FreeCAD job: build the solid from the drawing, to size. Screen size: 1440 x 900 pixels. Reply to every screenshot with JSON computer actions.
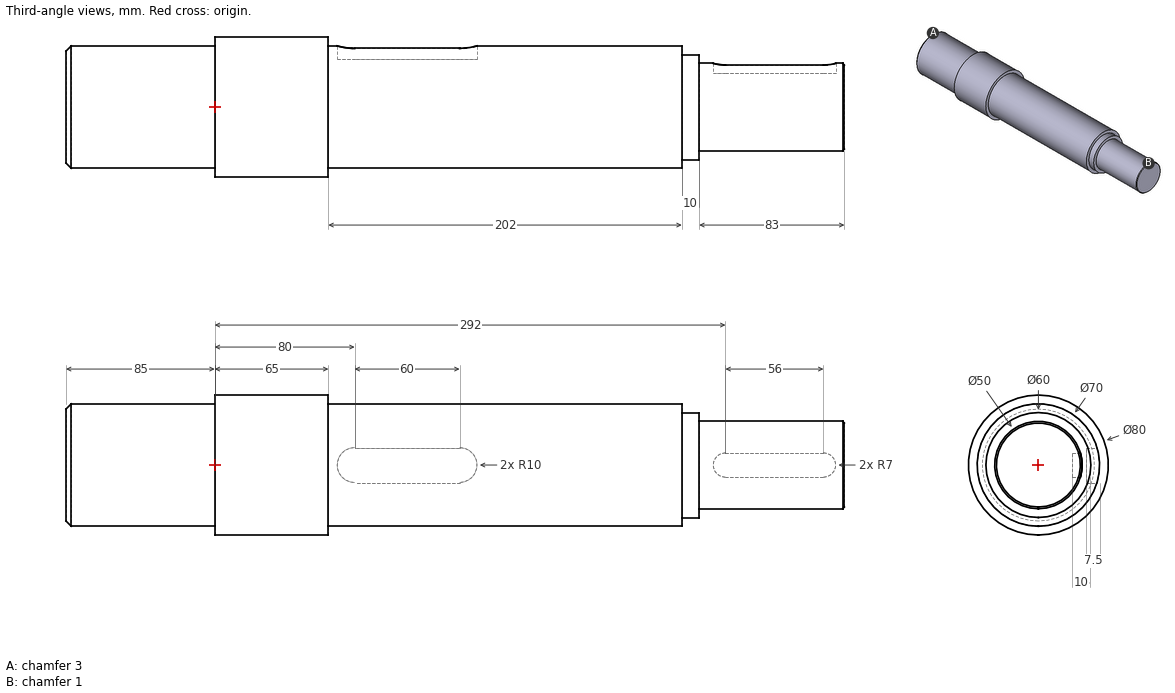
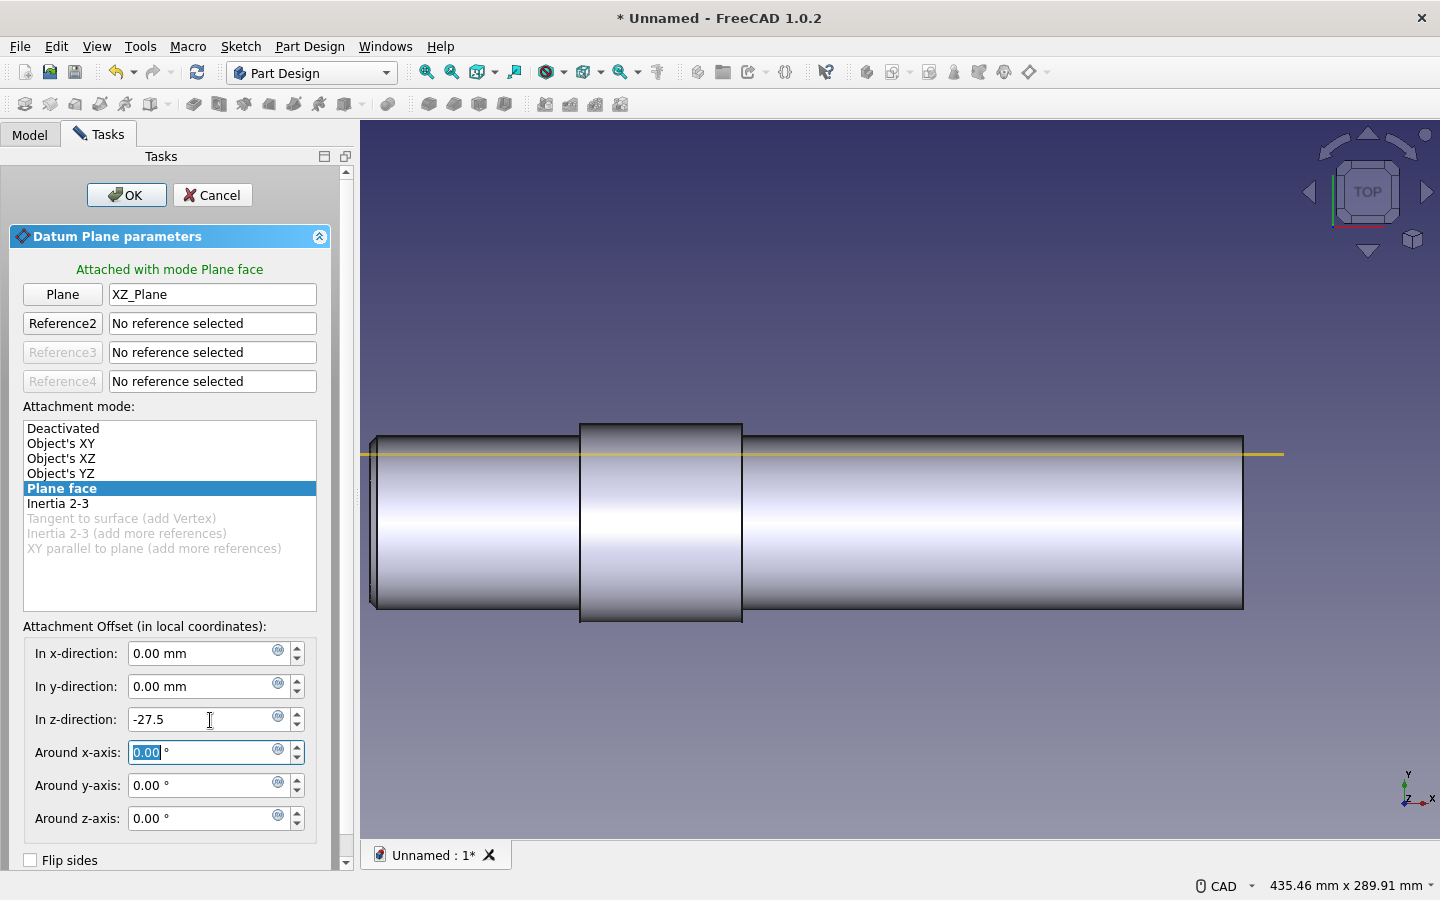
{"action": "left_click", "coordinate": [127, 195]}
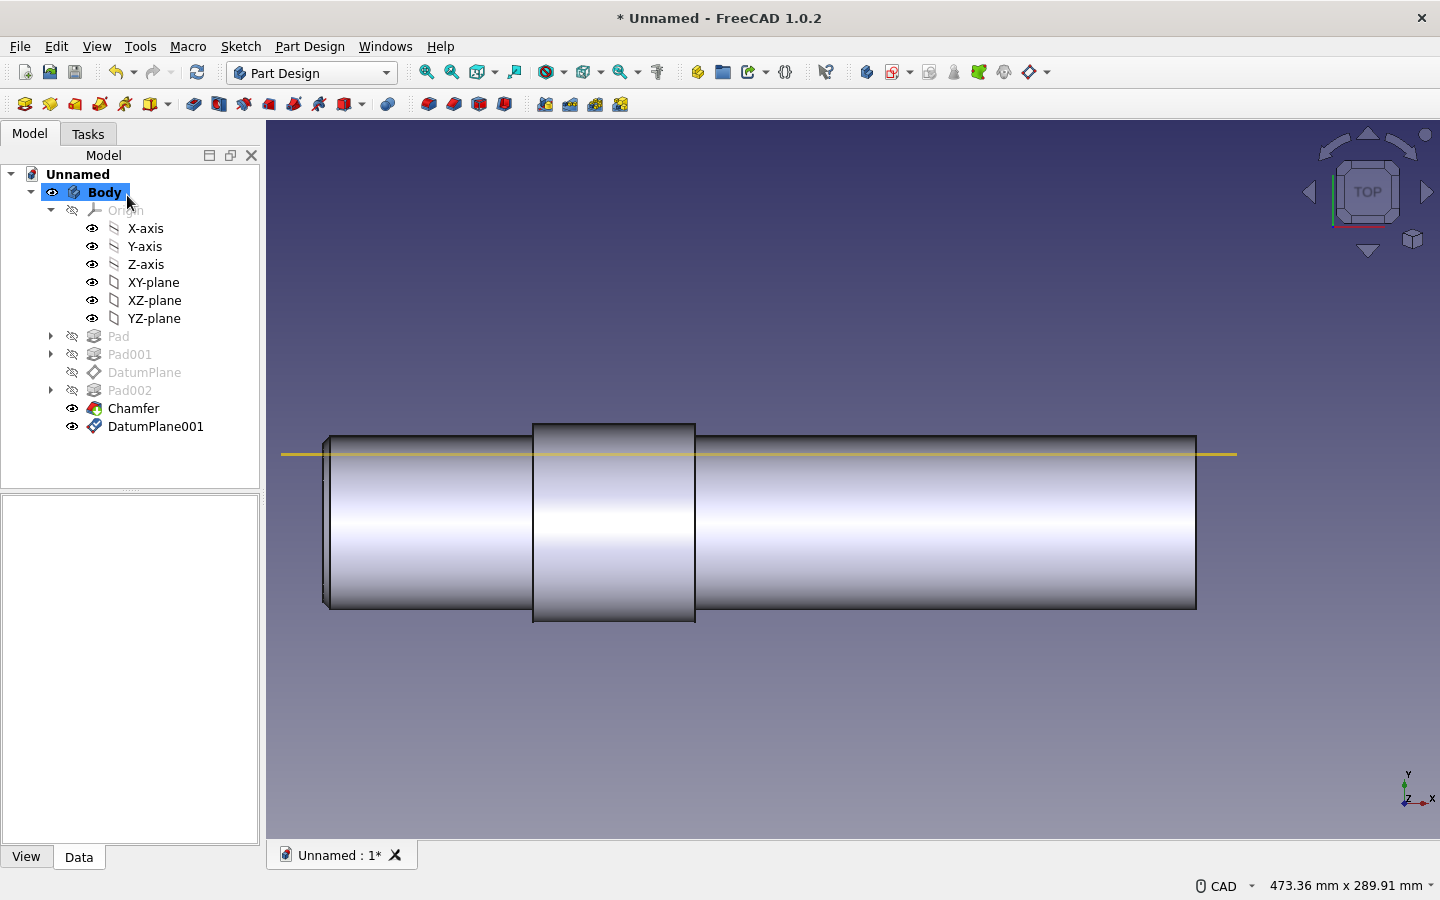
{"action": "left_click", "coordinate": [117, 426]}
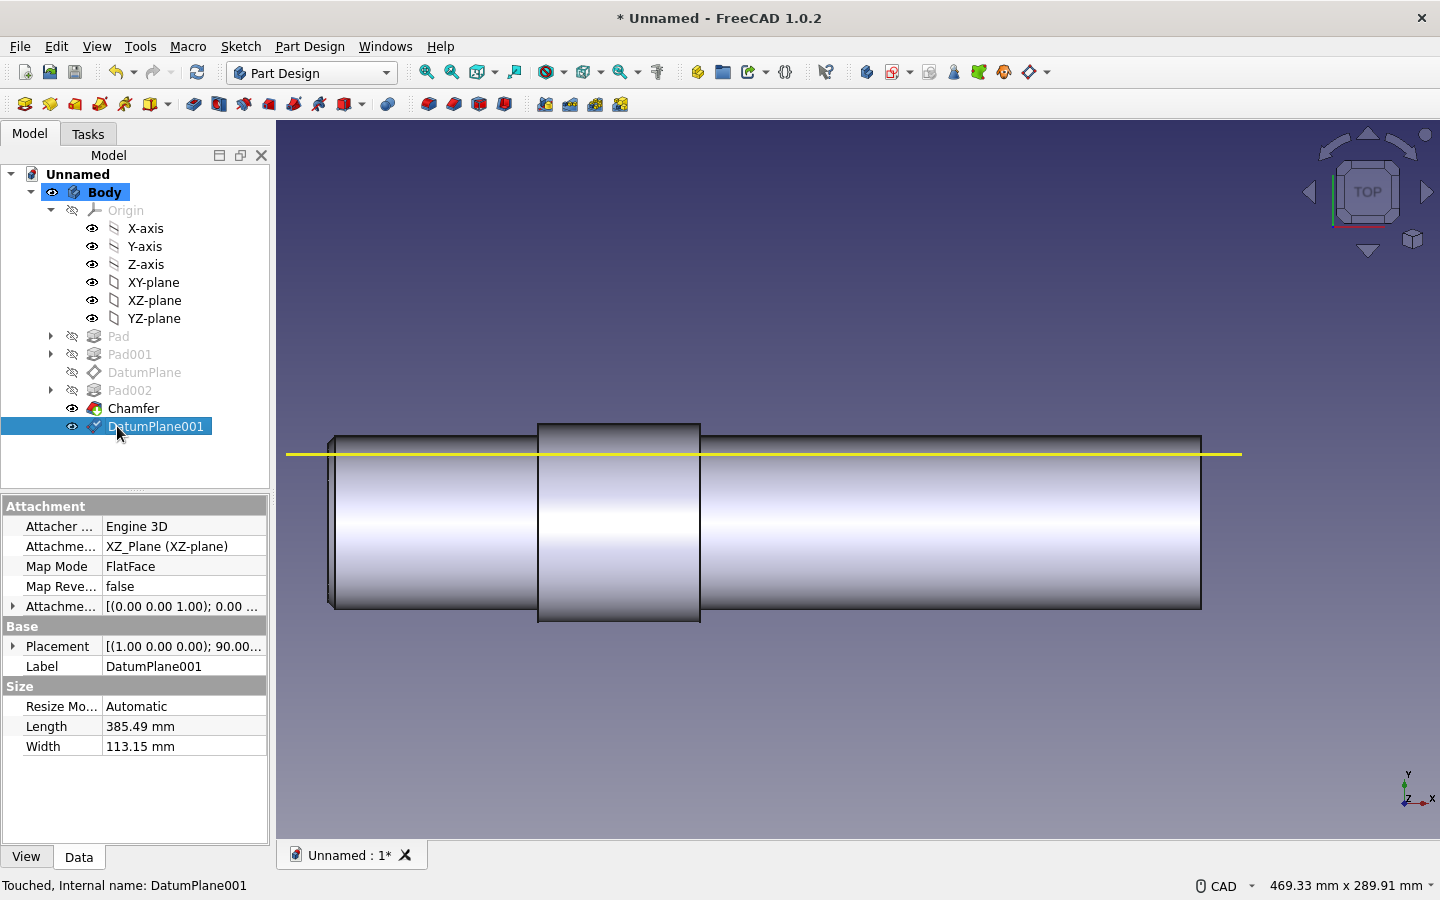
{"action": "left_click", "coordinate": [892, 72]}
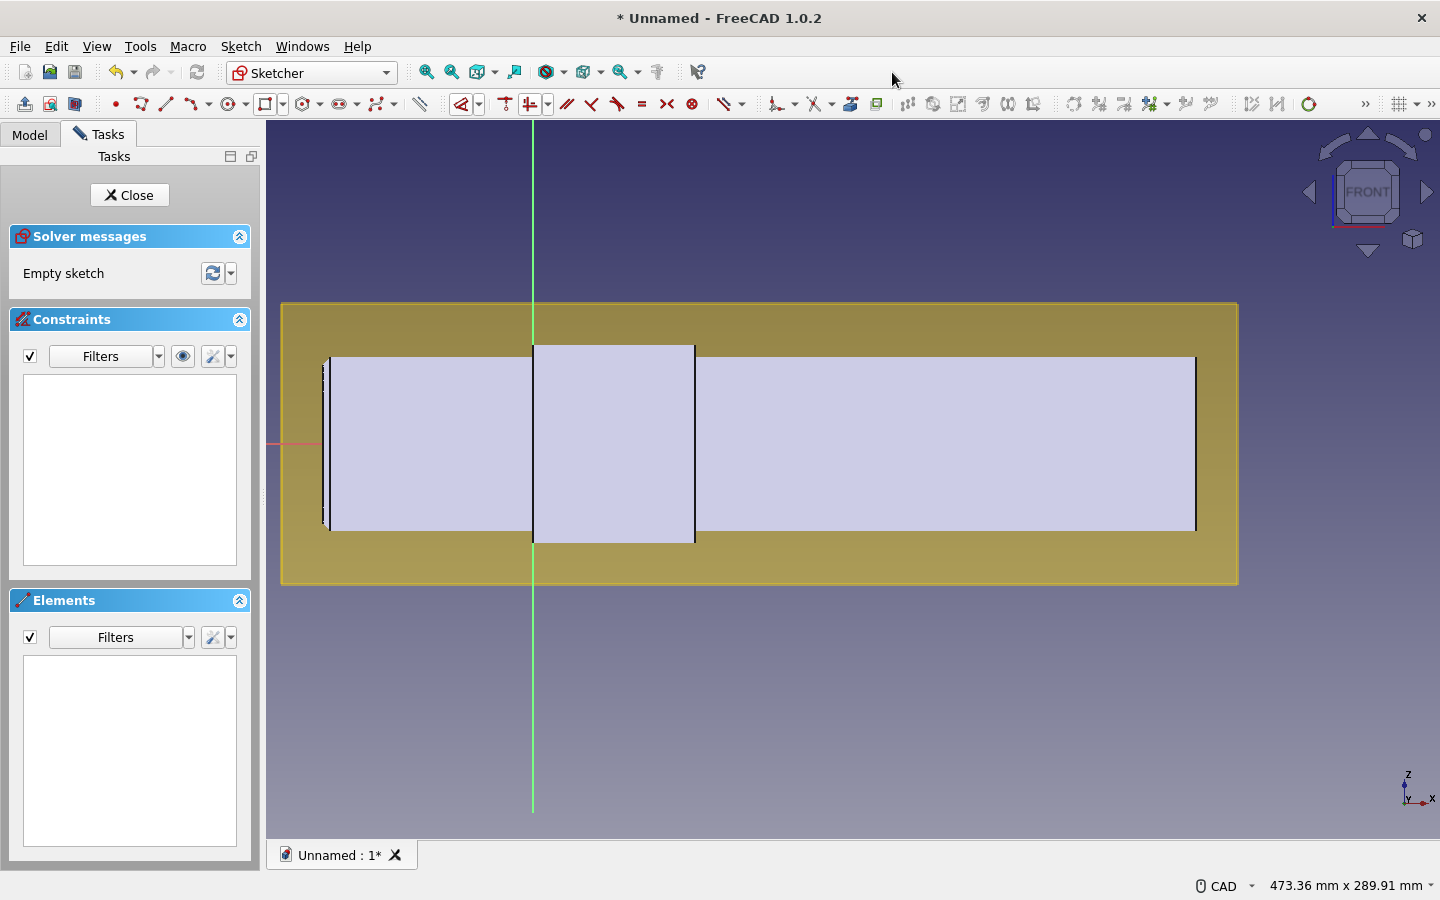
{"action": "left_click", "coordinate": [75, 104]}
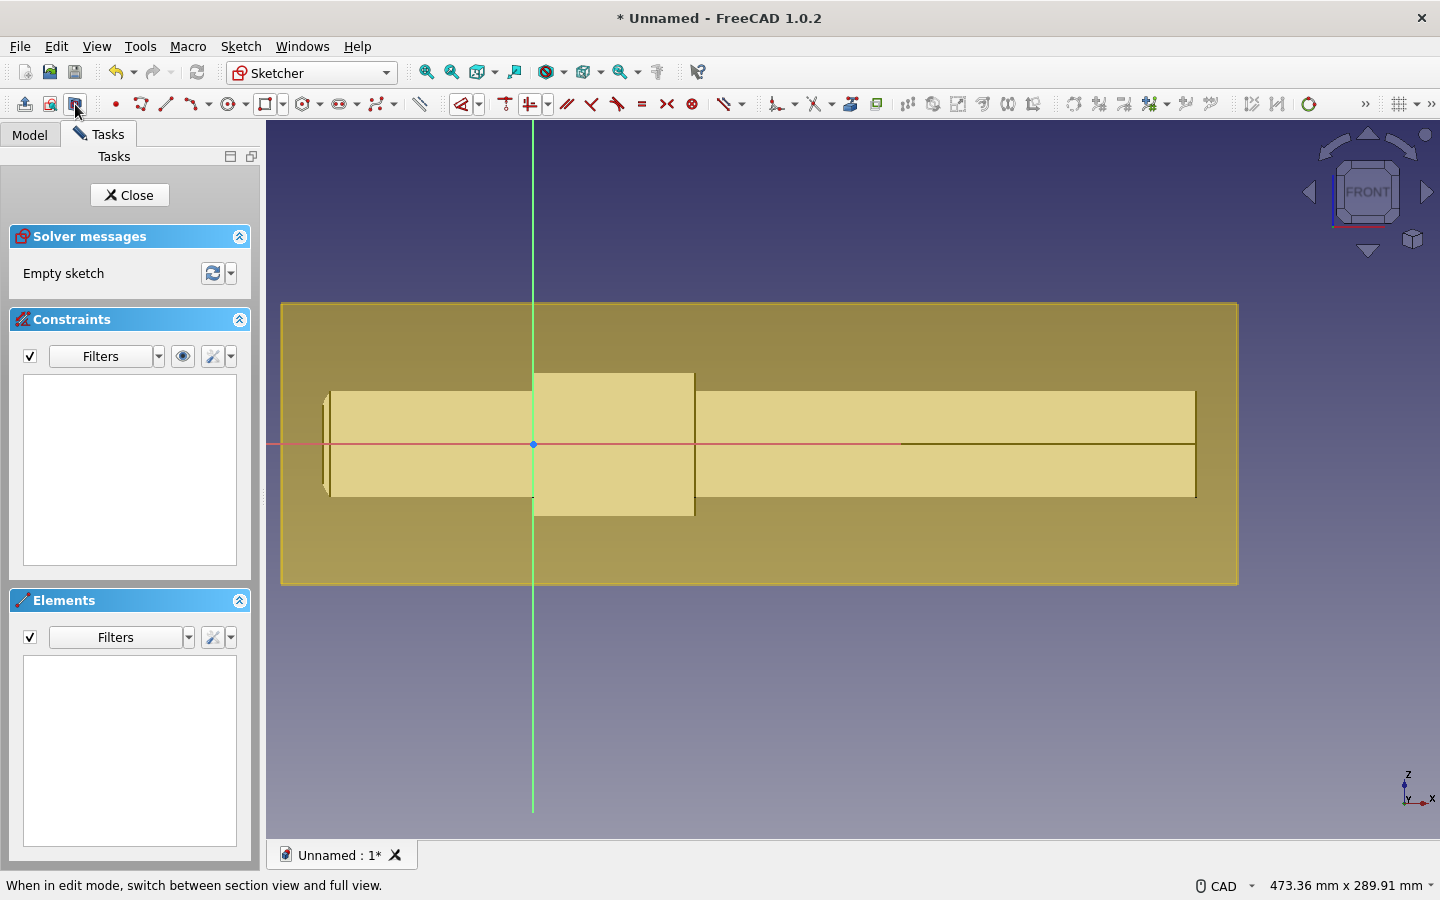
{"action": "scroll", "coordinate": [640, 401], "scroll_direction": "up", "scroll_amount": 3}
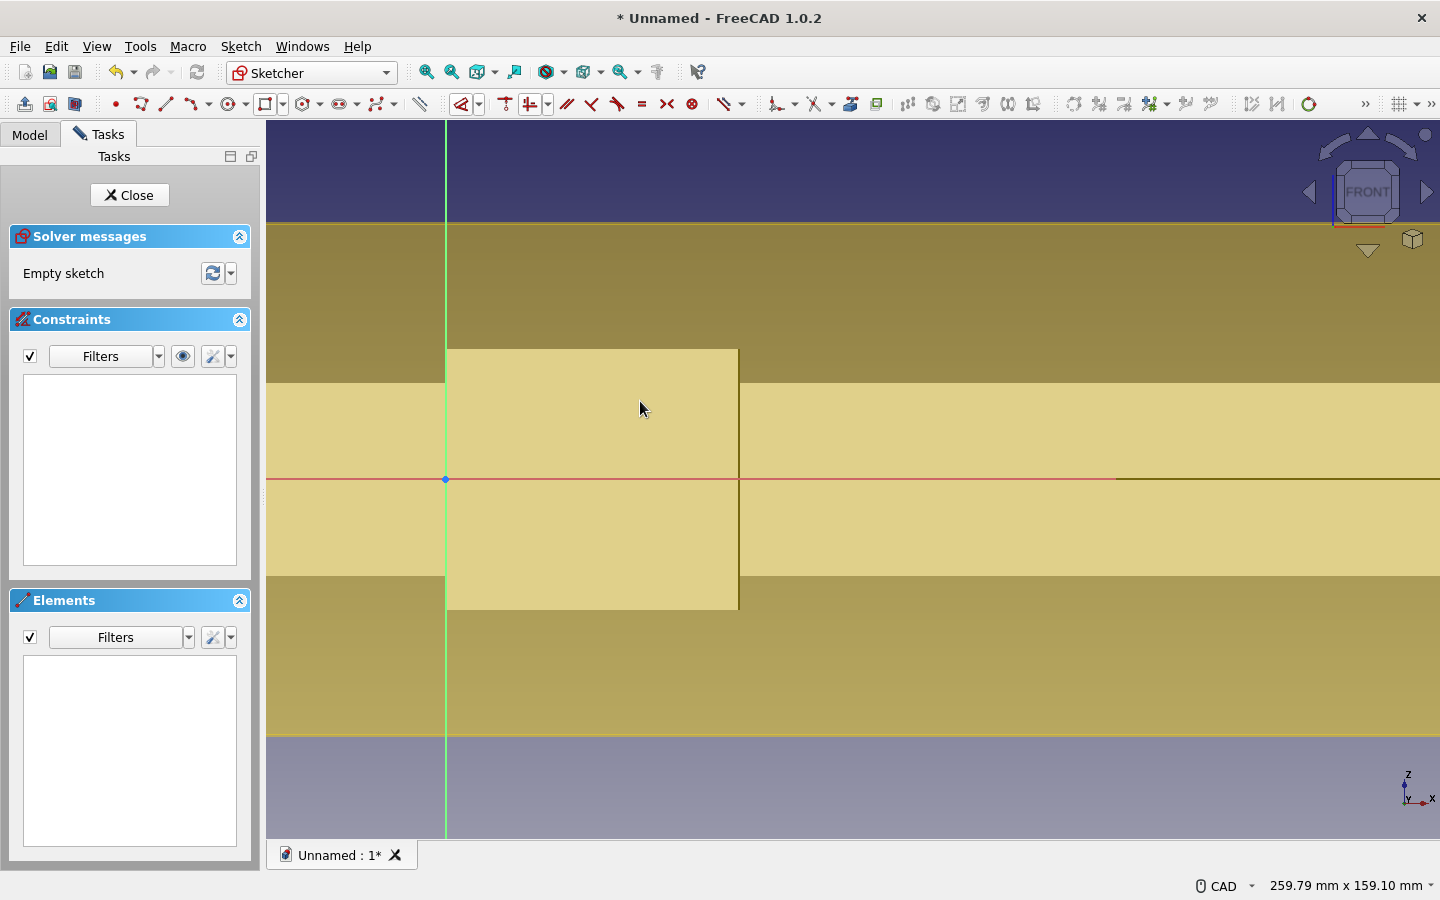
{"action": "key", "text": "g s"}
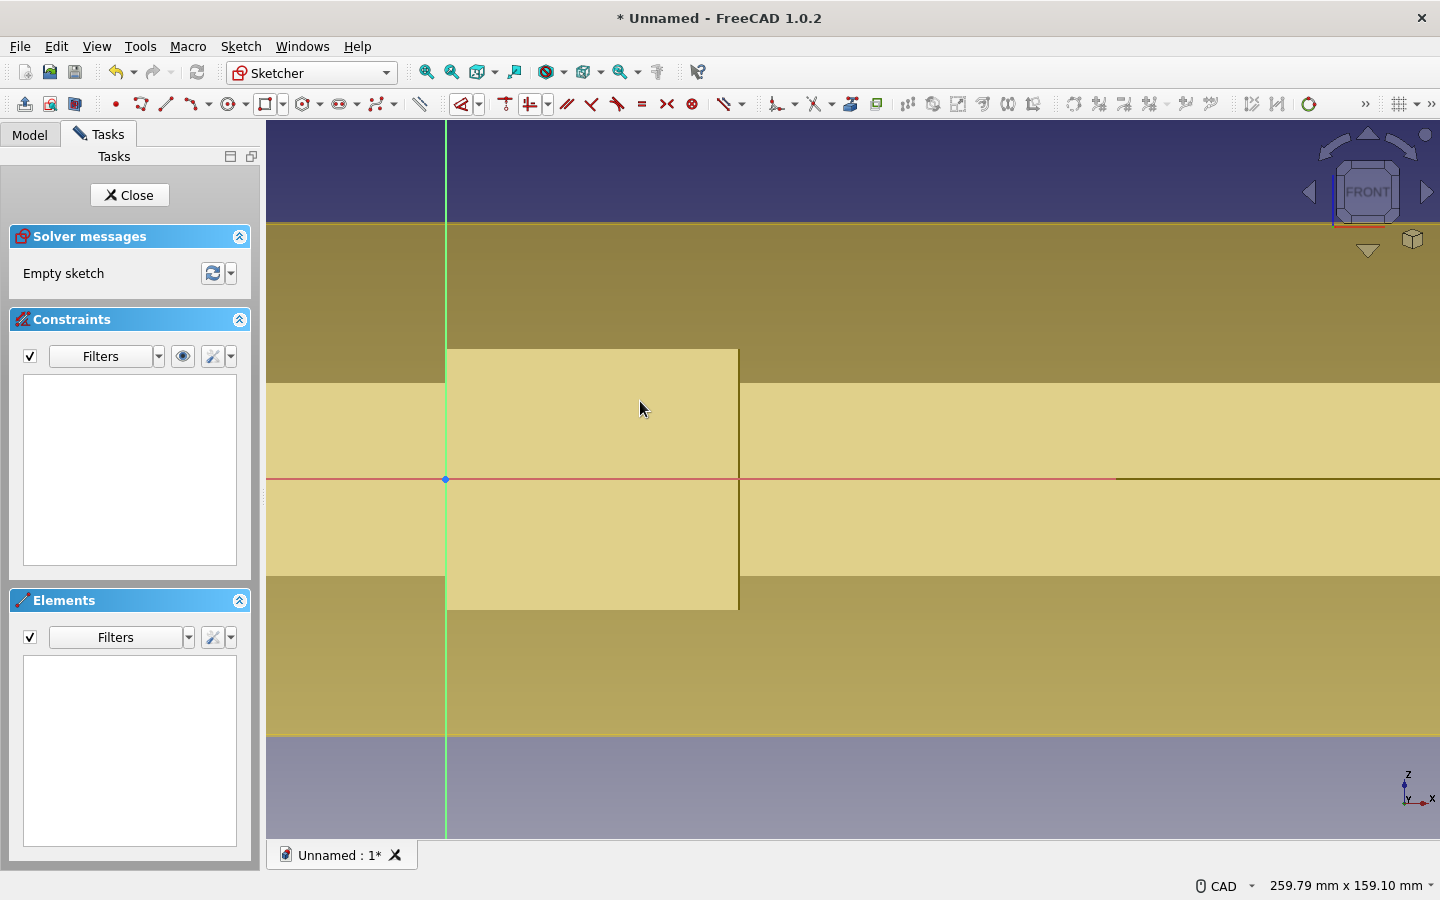
{"action": "left_click", "coordinate": [807, 479]}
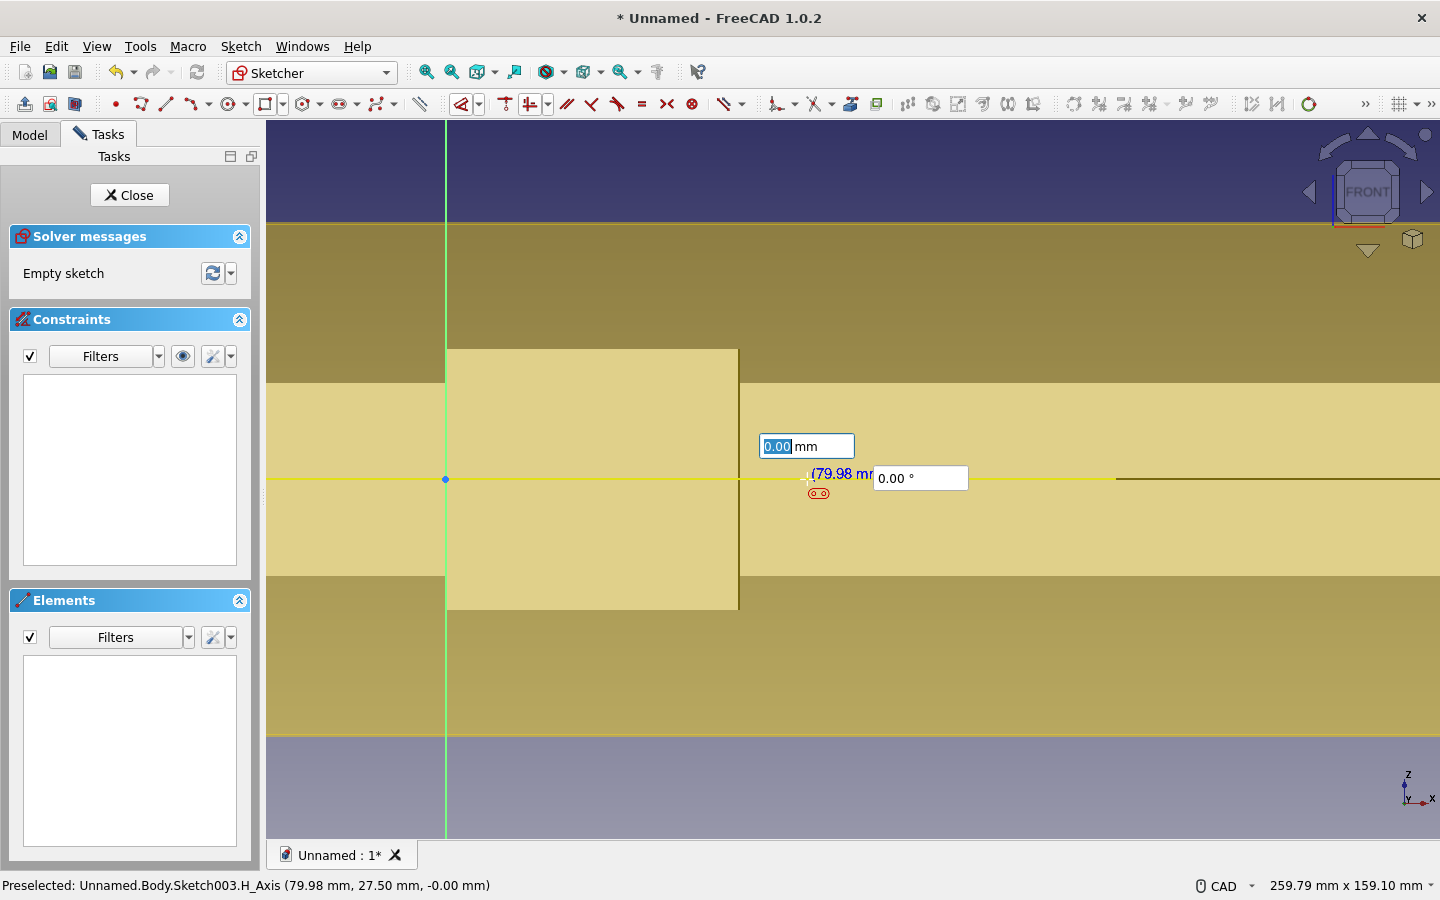
{"action": "left_click", "coordinate": [1078, 470]}